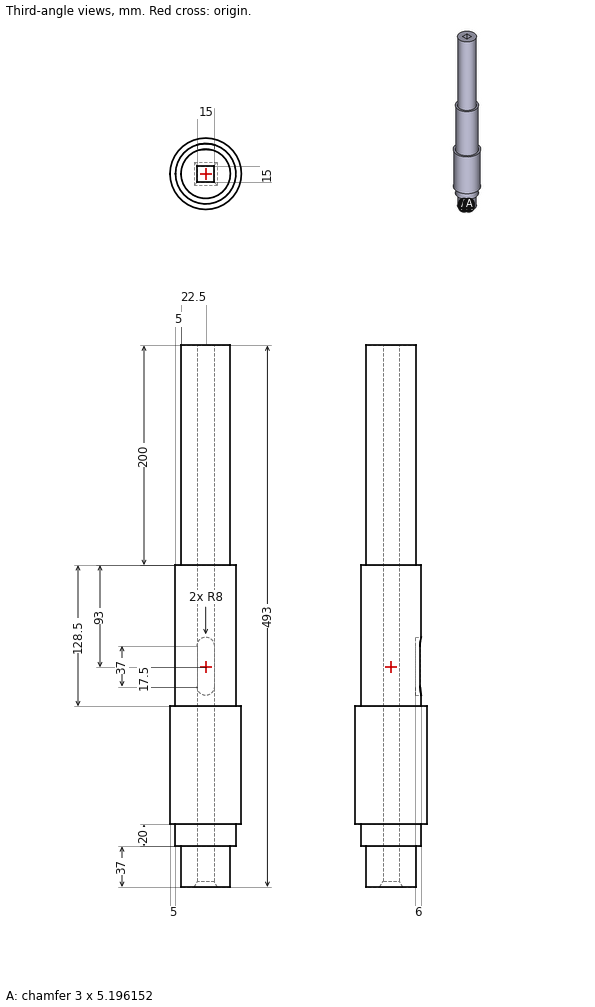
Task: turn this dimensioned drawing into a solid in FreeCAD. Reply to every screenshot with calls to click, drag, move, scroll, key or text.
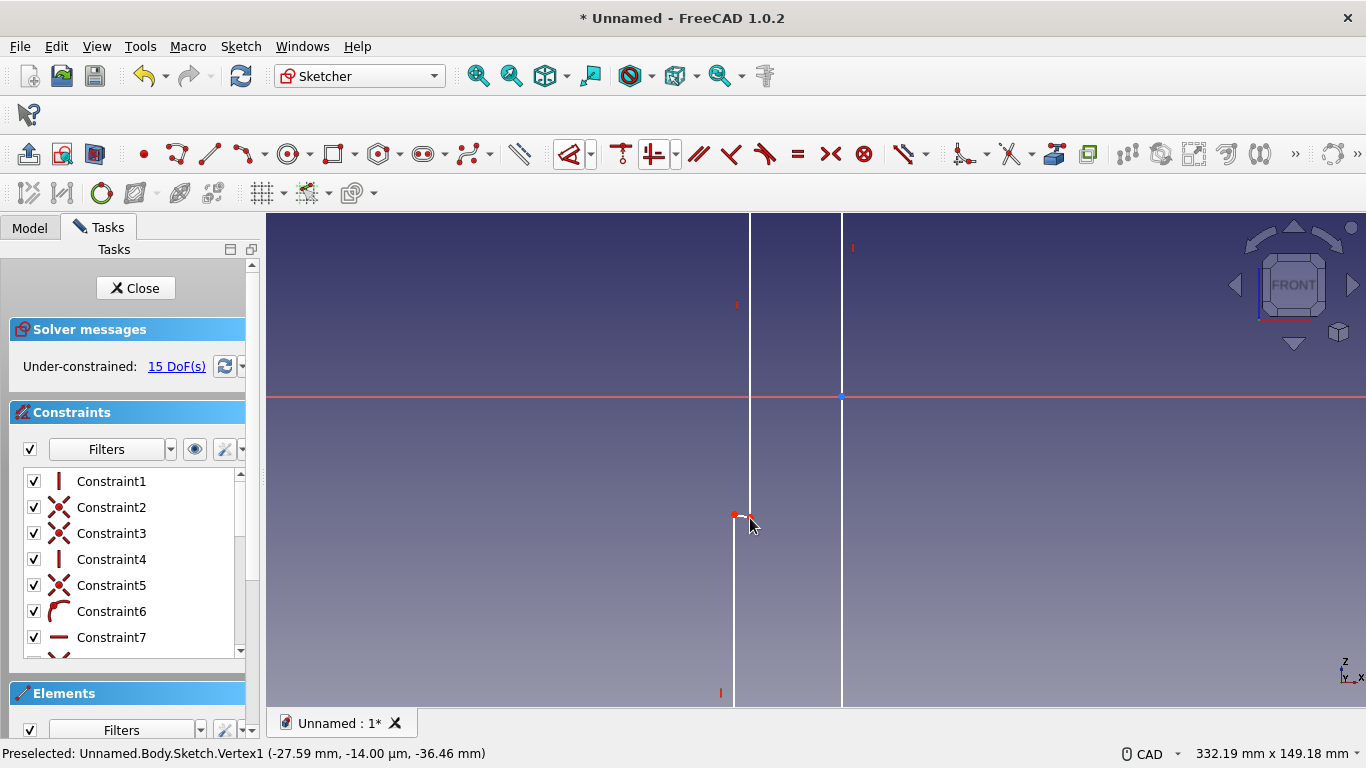
scroll(737, 515, down, 8)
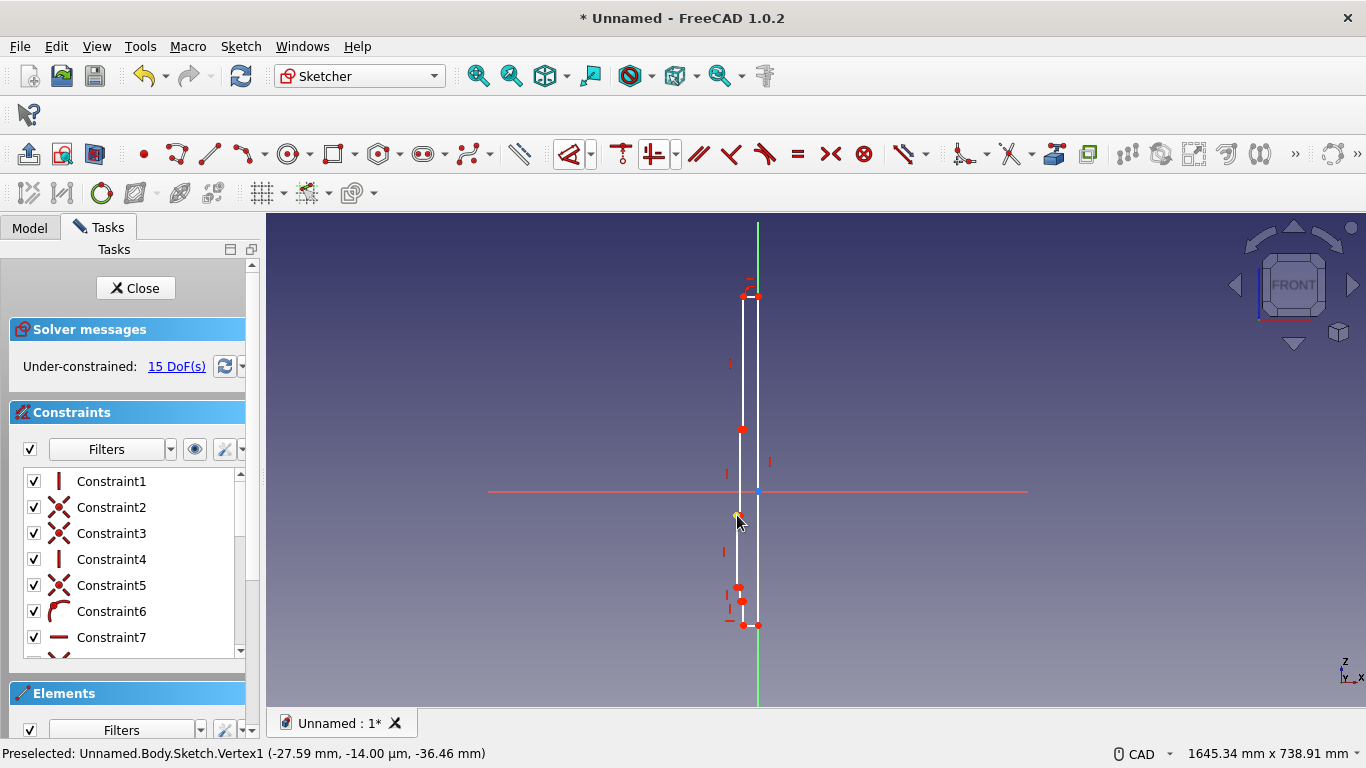
scroll(742, 430, up, 11)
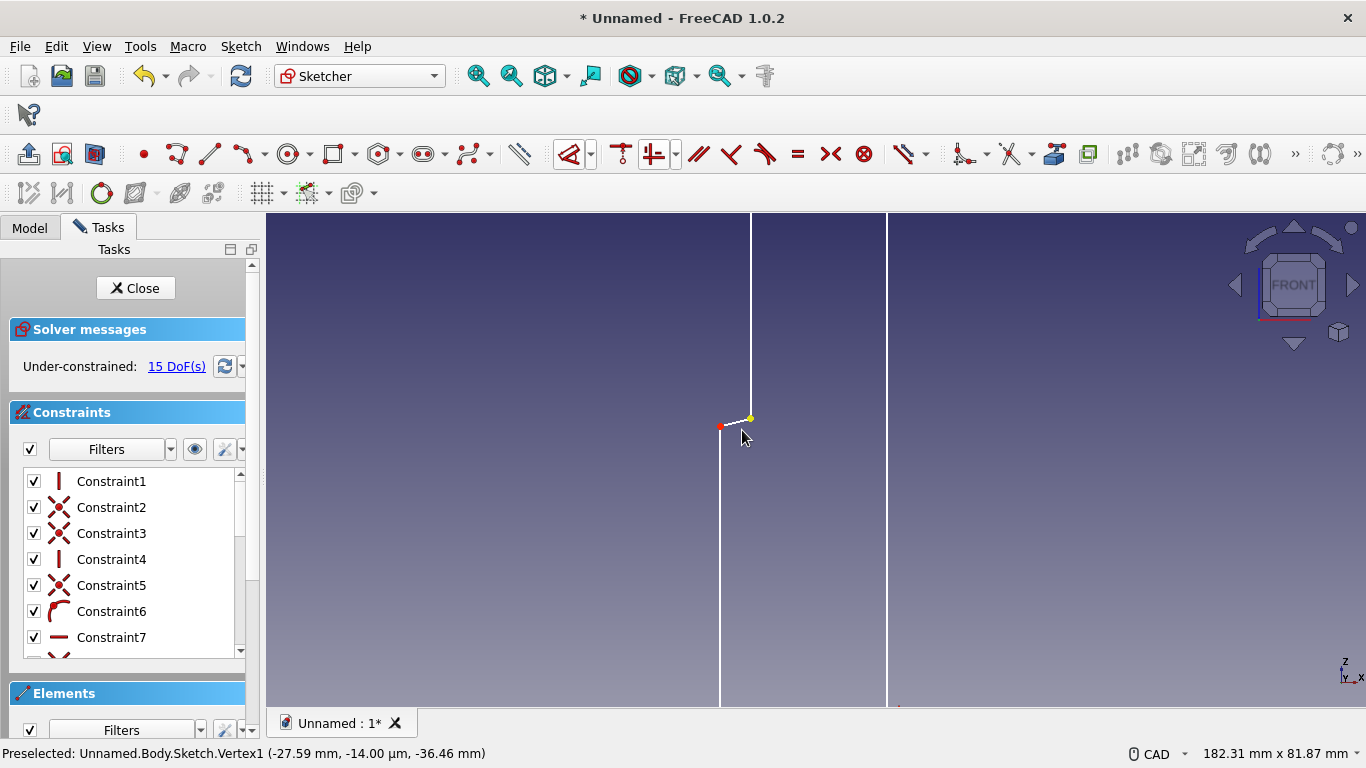
click(736, 423)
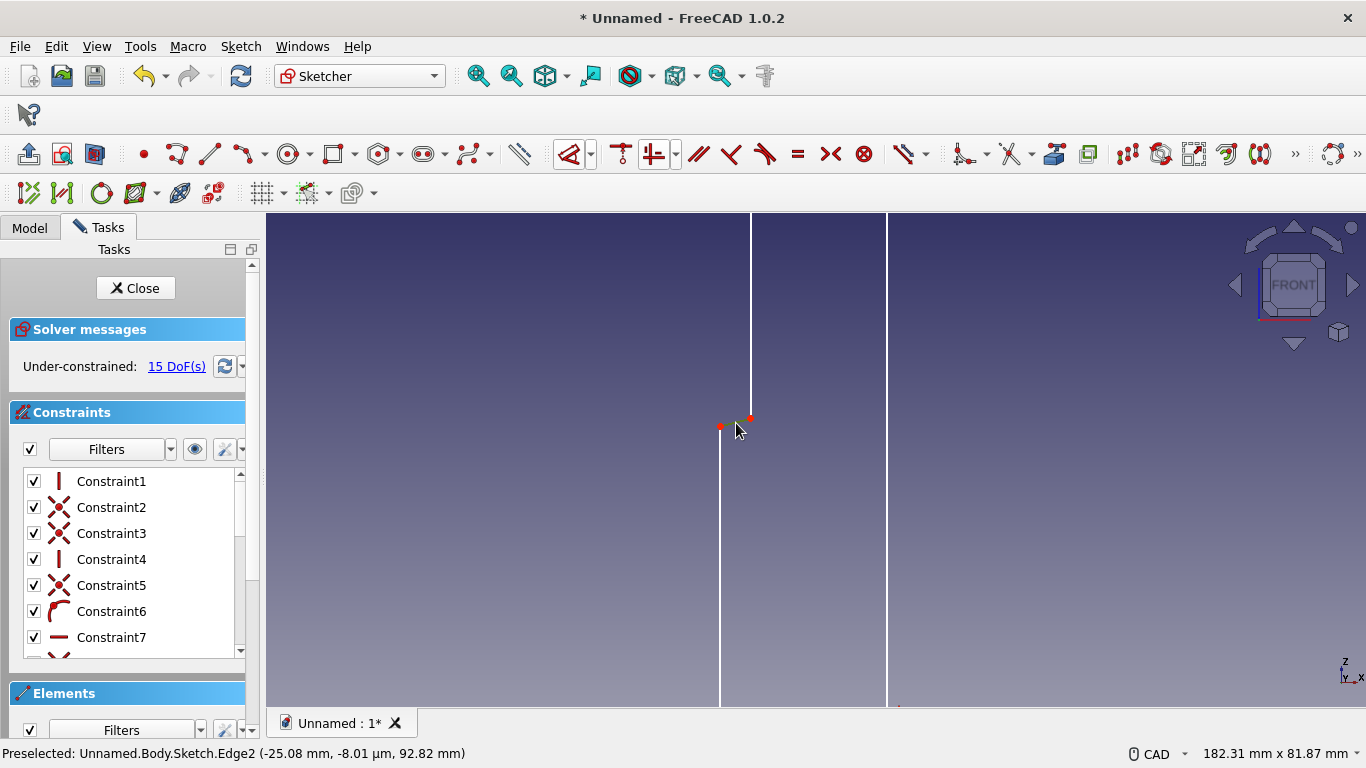
key(h)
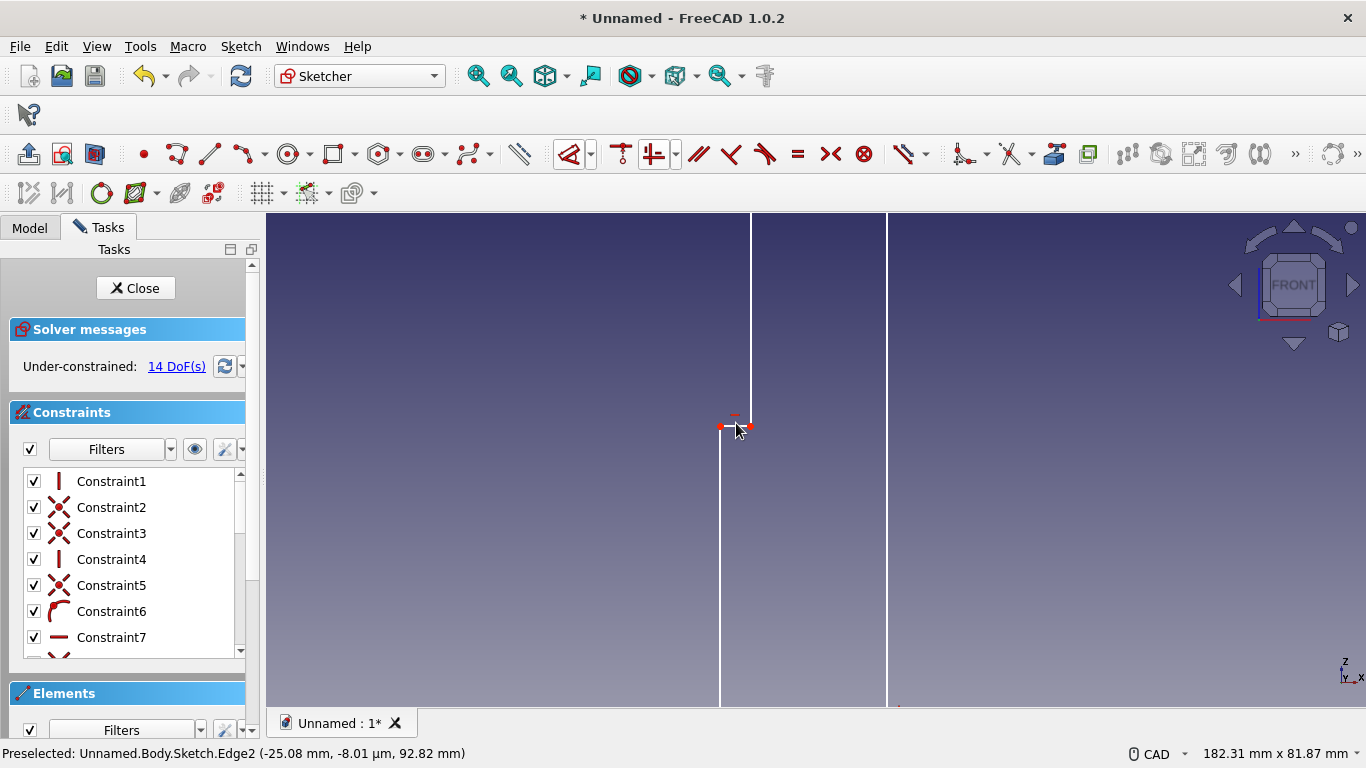
scroll(742, 430, down, 11)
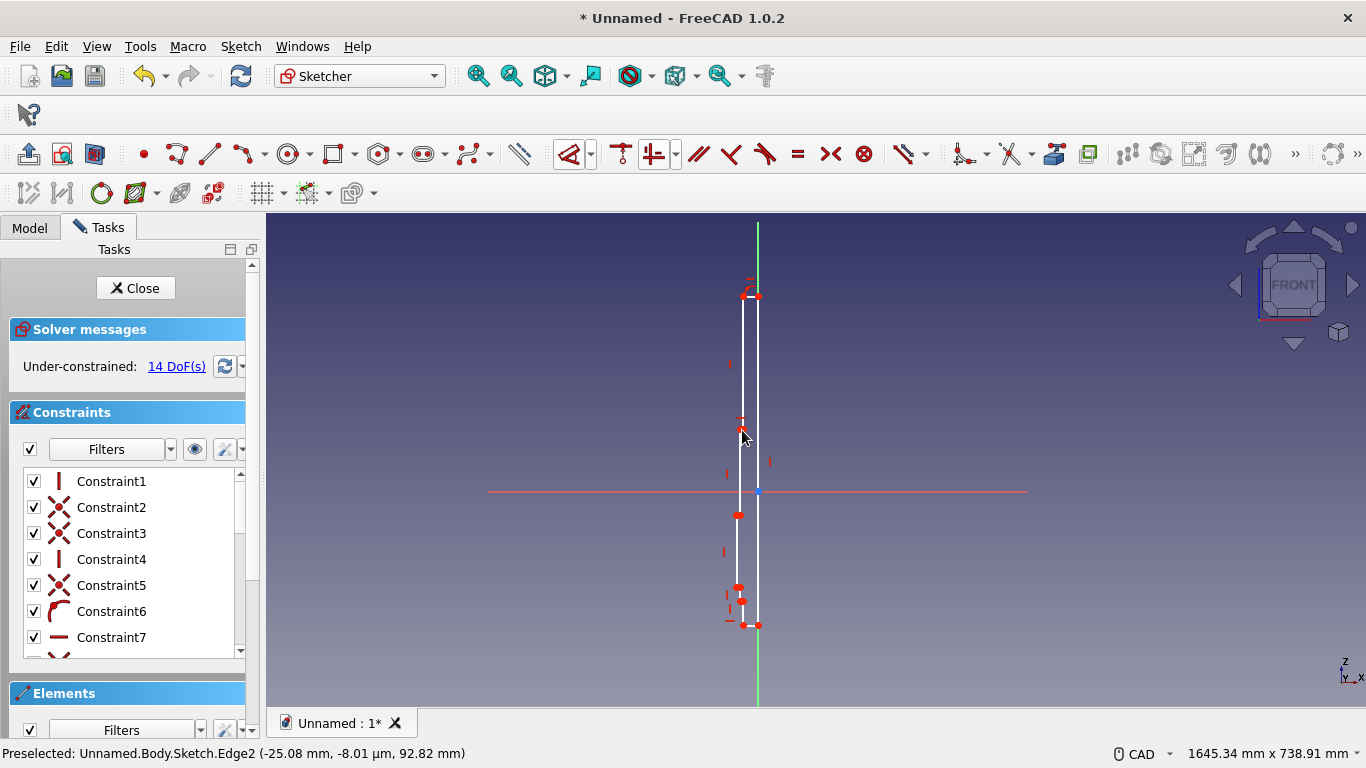
scroll(742, 602, up, 13)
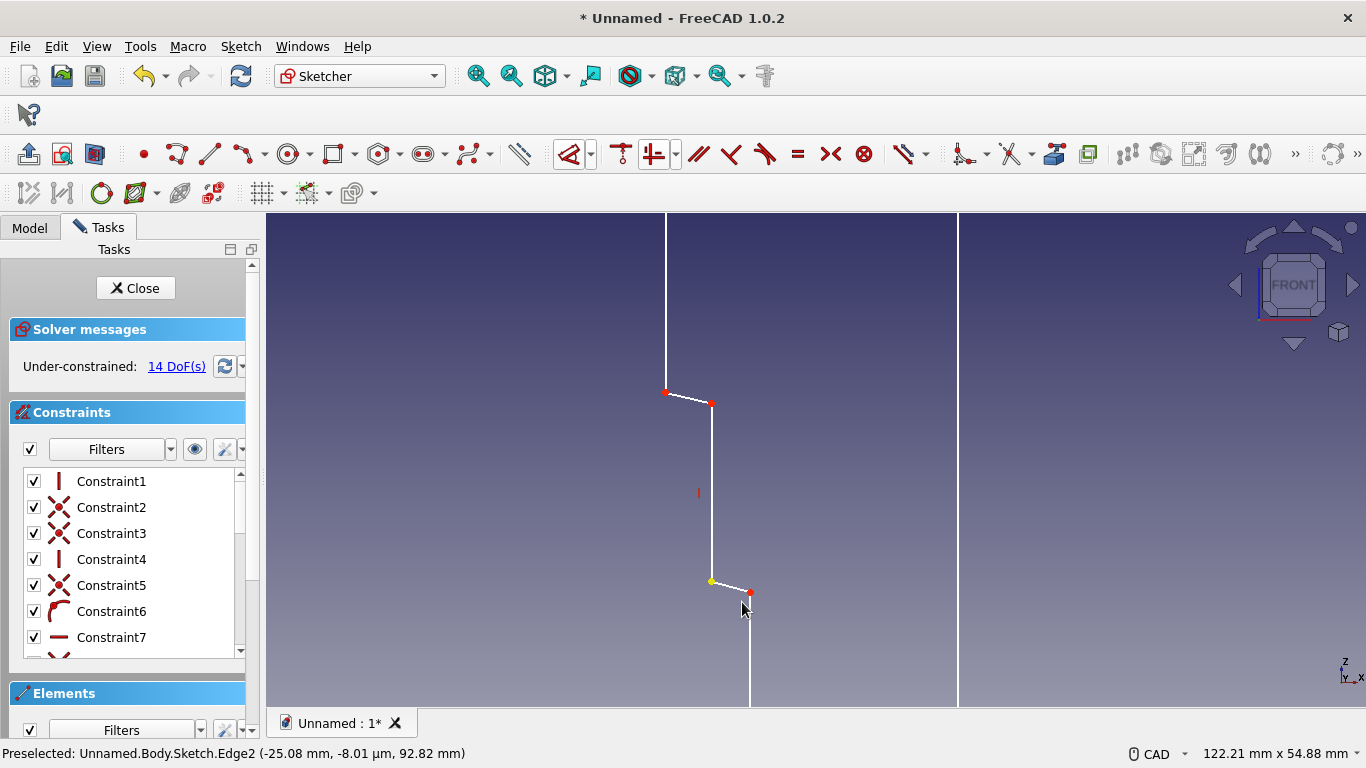
click(735, 588)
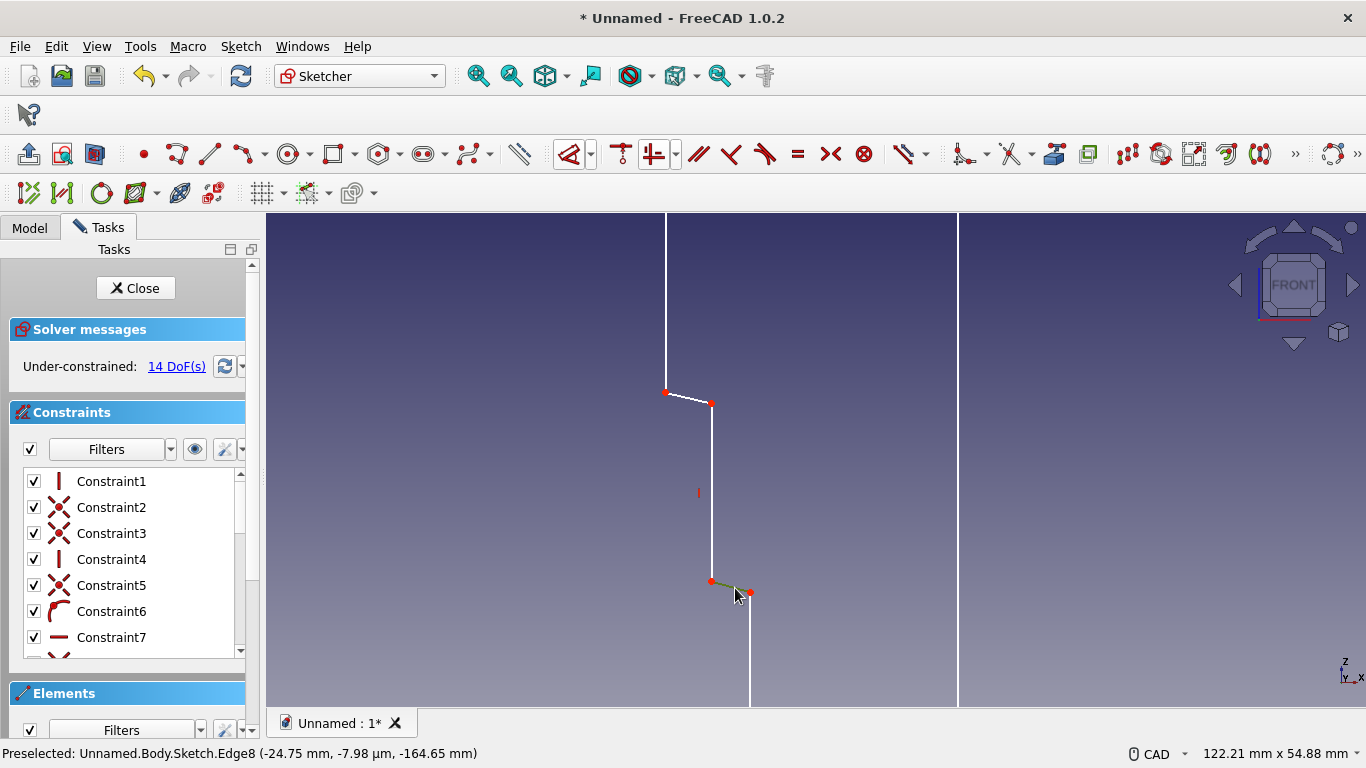
click(676, 154)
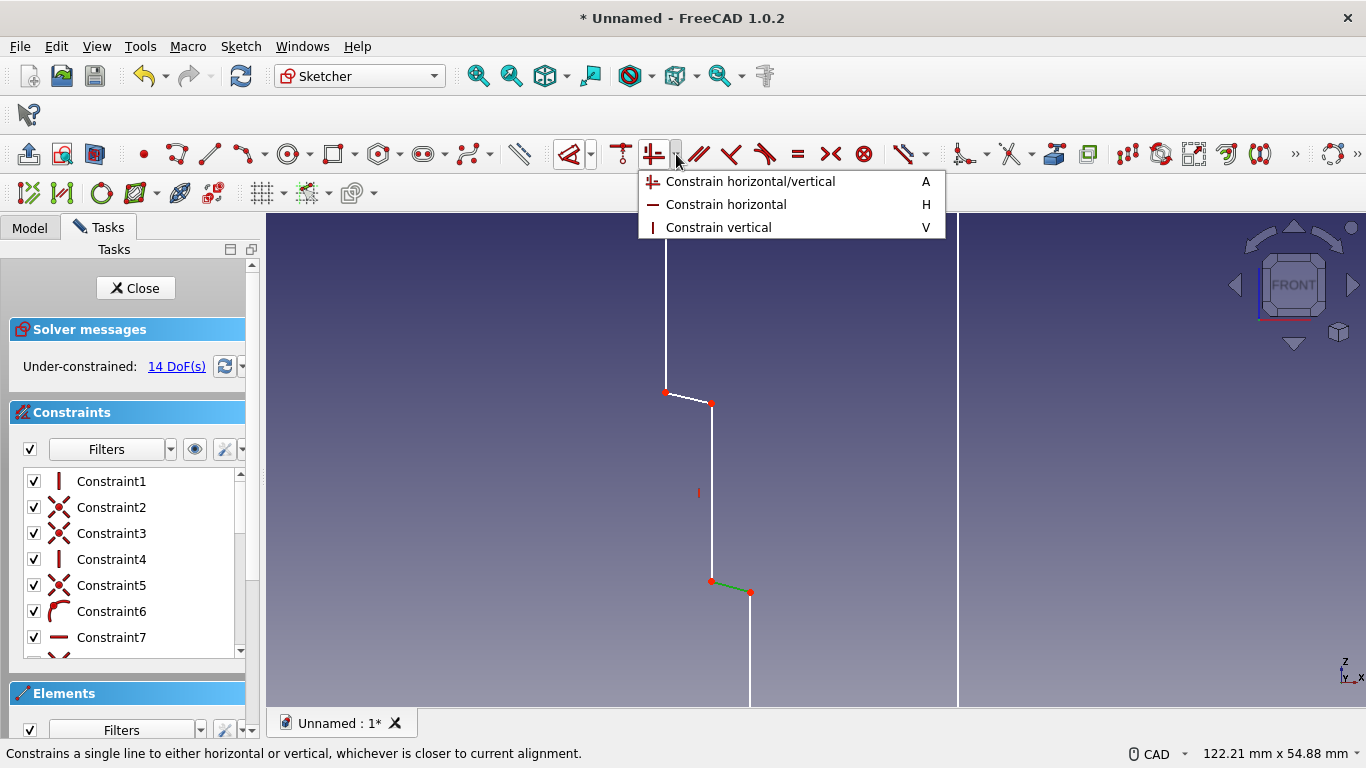
click(792, 204)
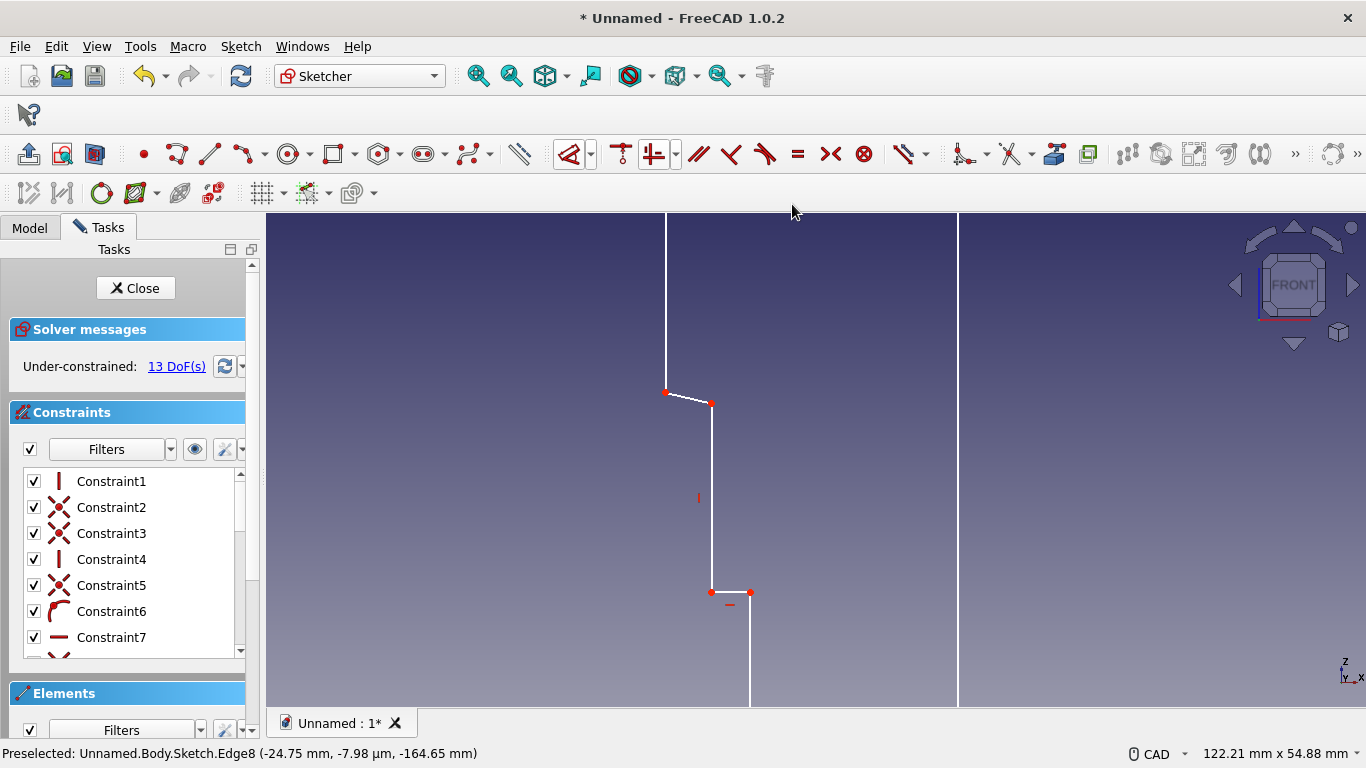
click(698, 400)